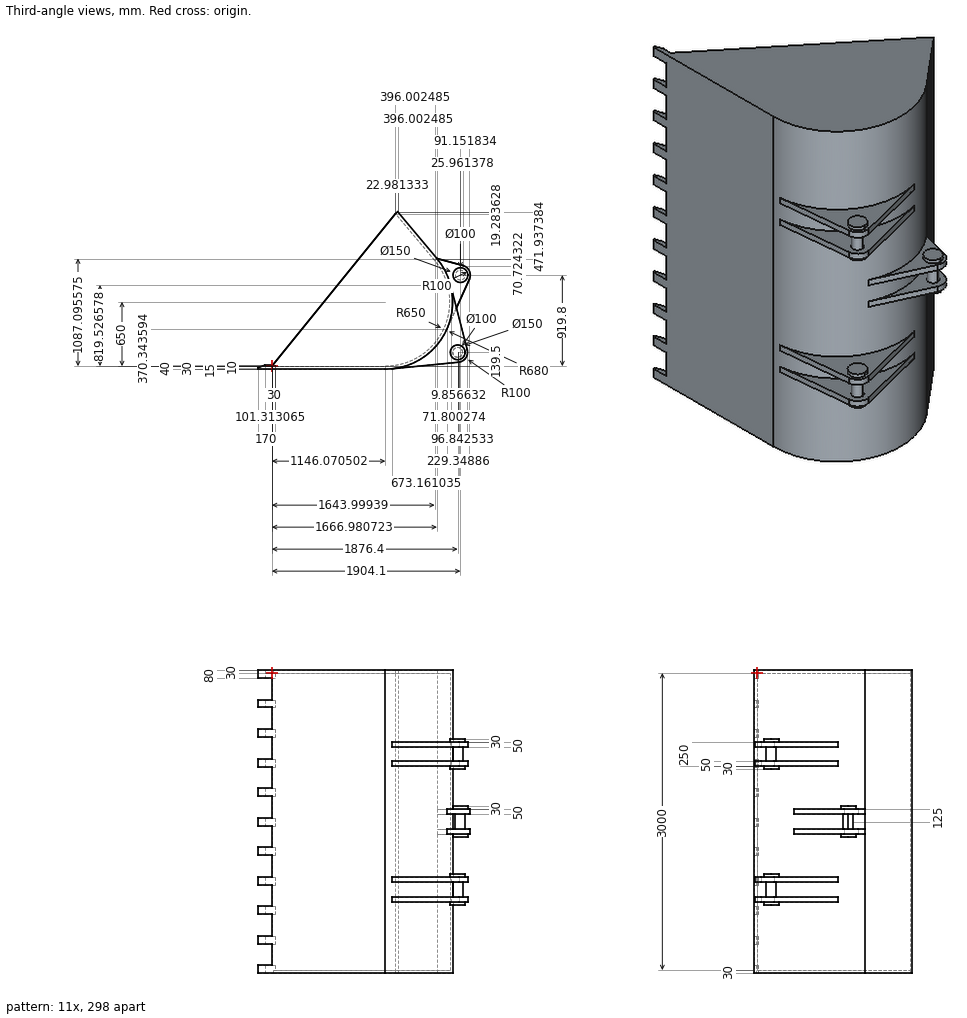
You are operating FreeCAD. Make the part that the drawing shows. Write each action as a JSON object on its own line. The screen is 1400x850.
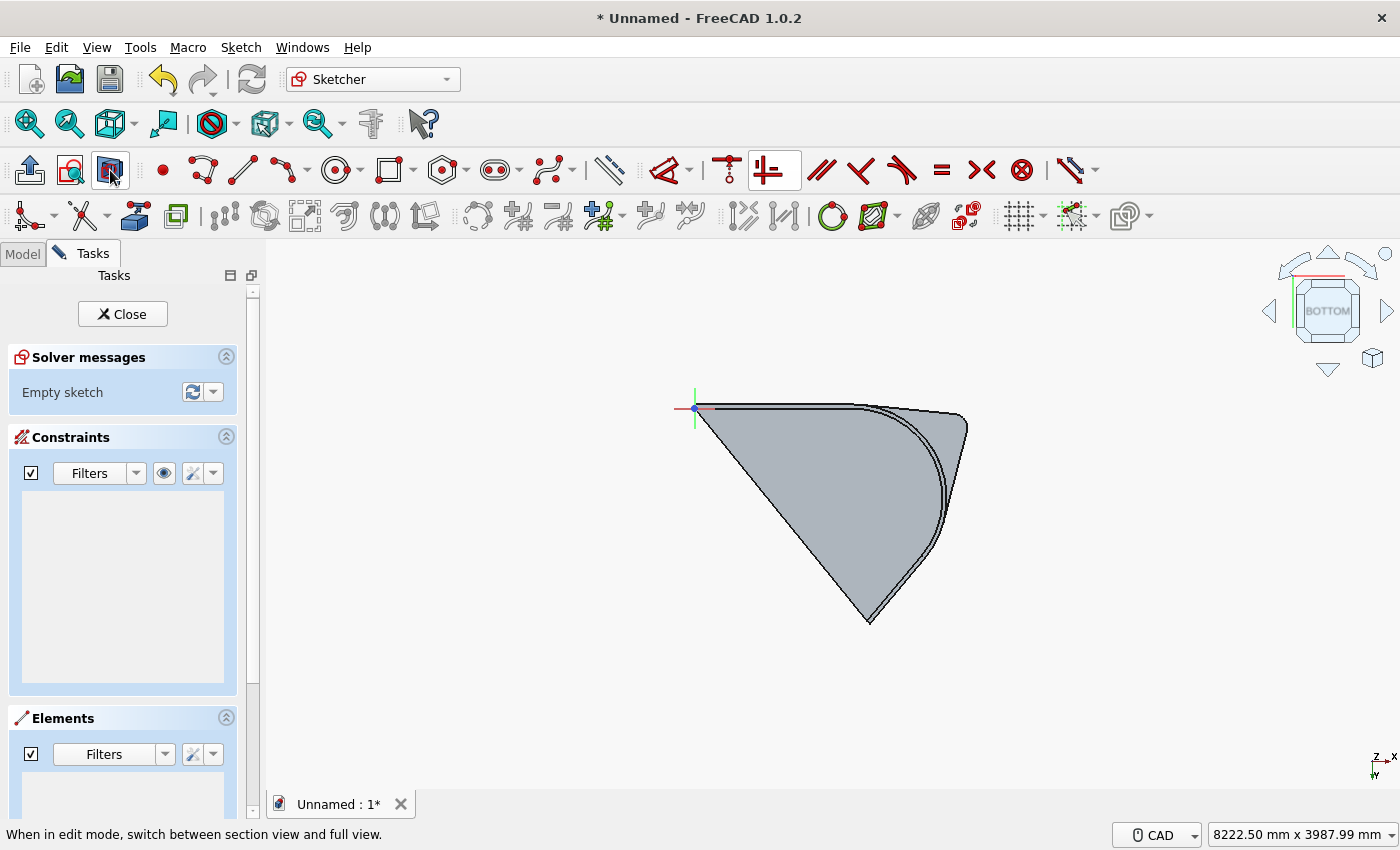
{"action": "scroll", "coordinate": [966, 422], "scroll_direction": "up", "scroll_amount": 14}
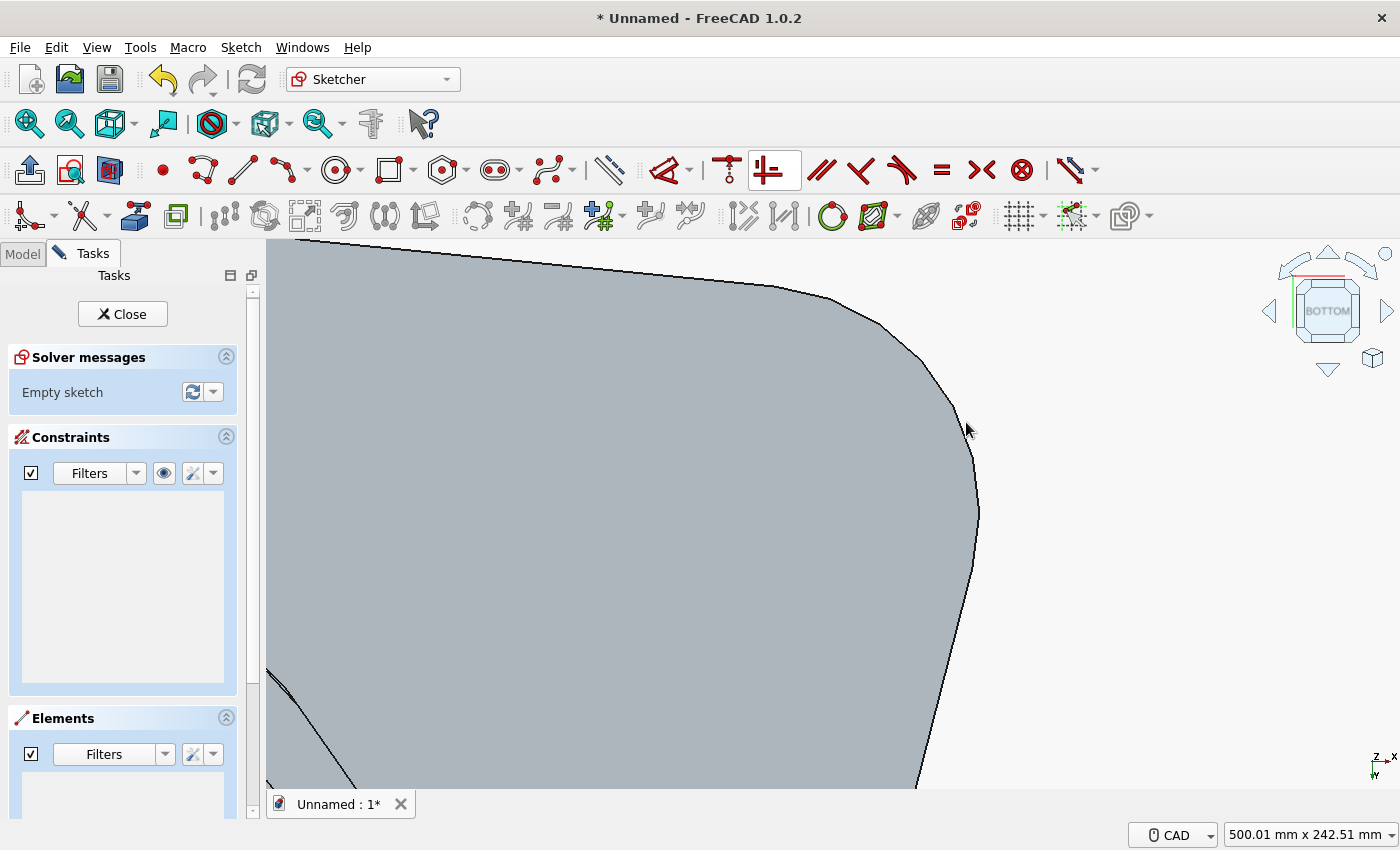
{"action": "key", "text": "g c"}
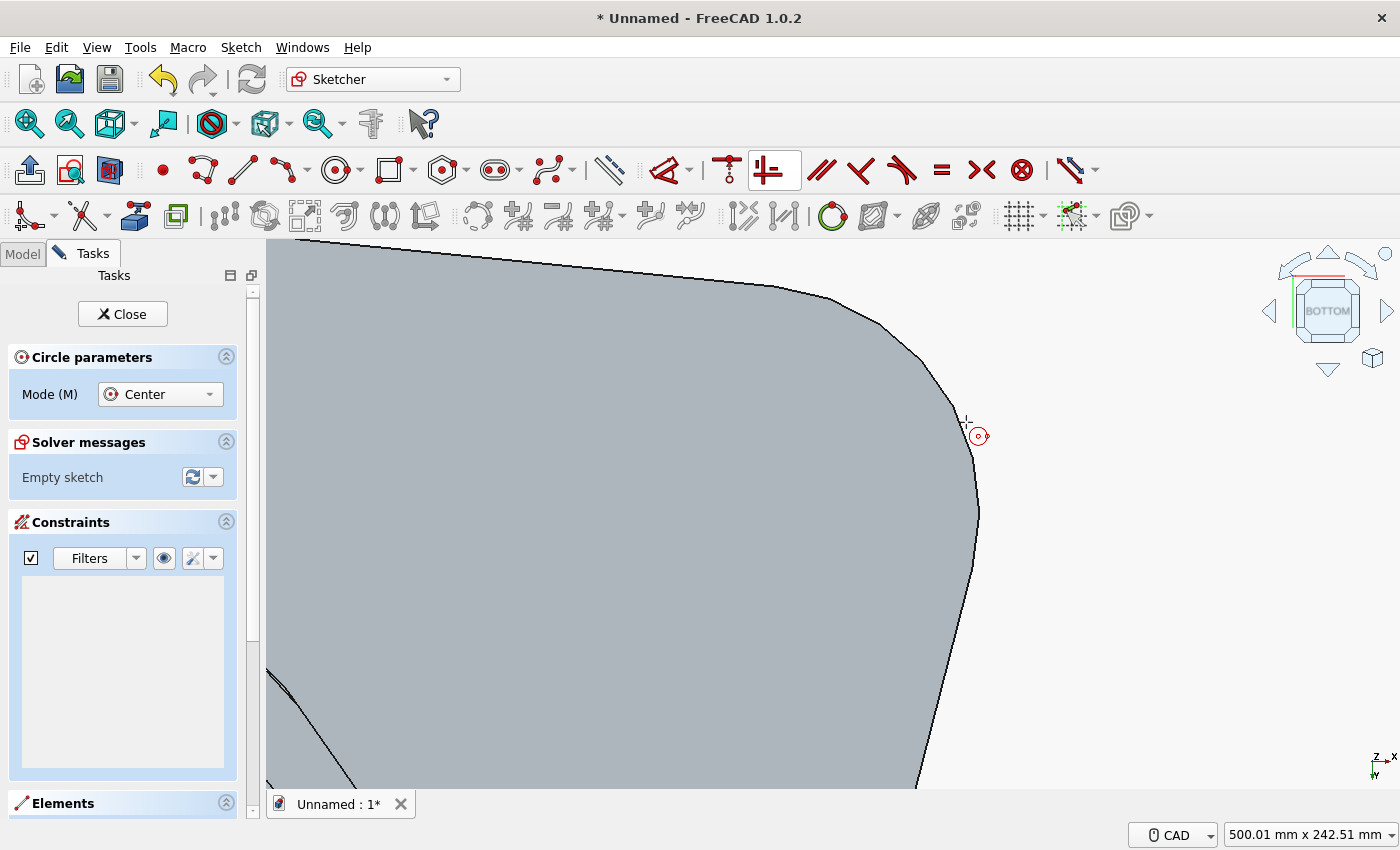
{"action": "left_click", "coordinate": [753, 512]}
{"action": "left_click", "coordinate": [873, 392]}
{"action": "key", "text": "Escape"}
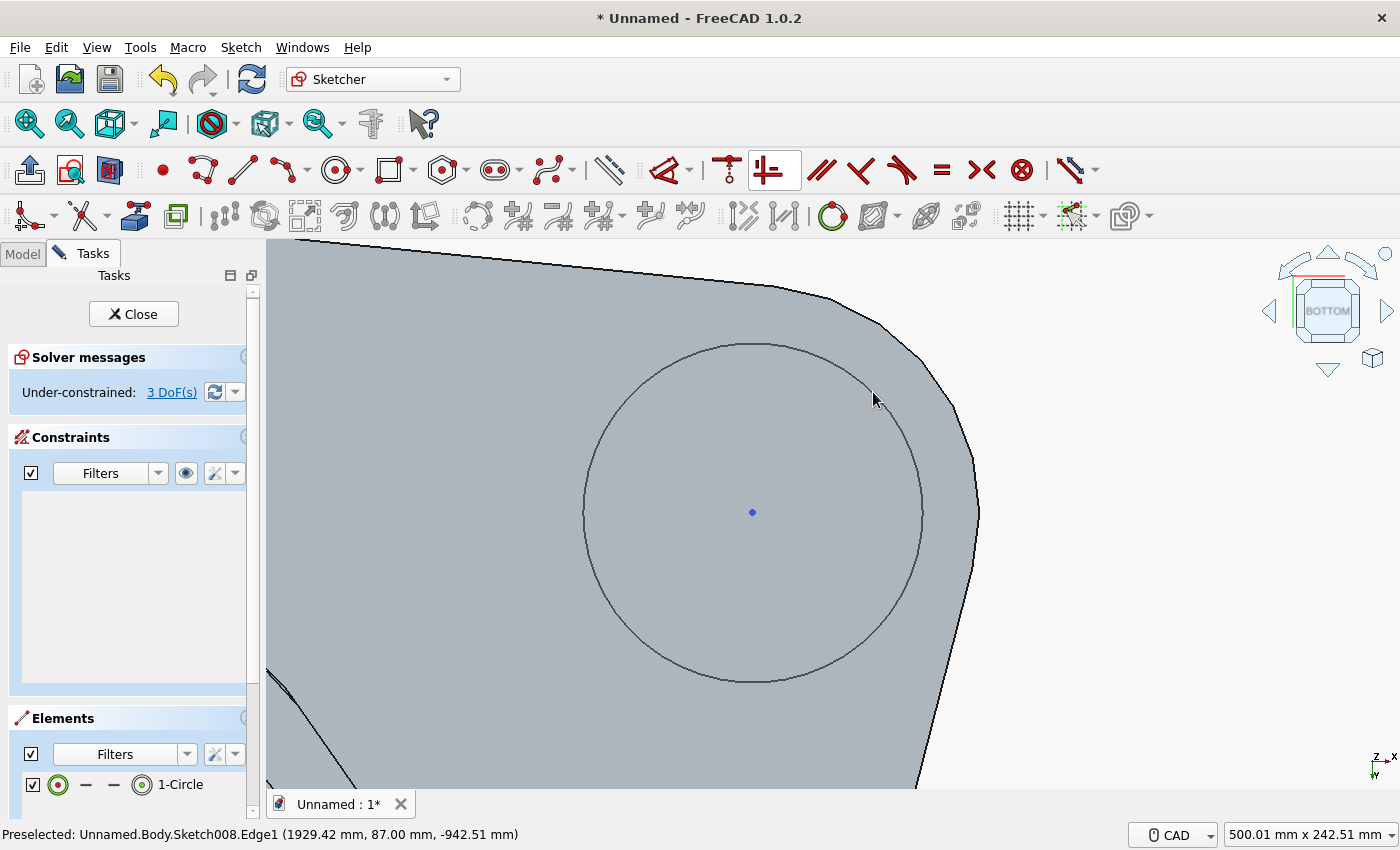
{"action": "key", "text": "d"}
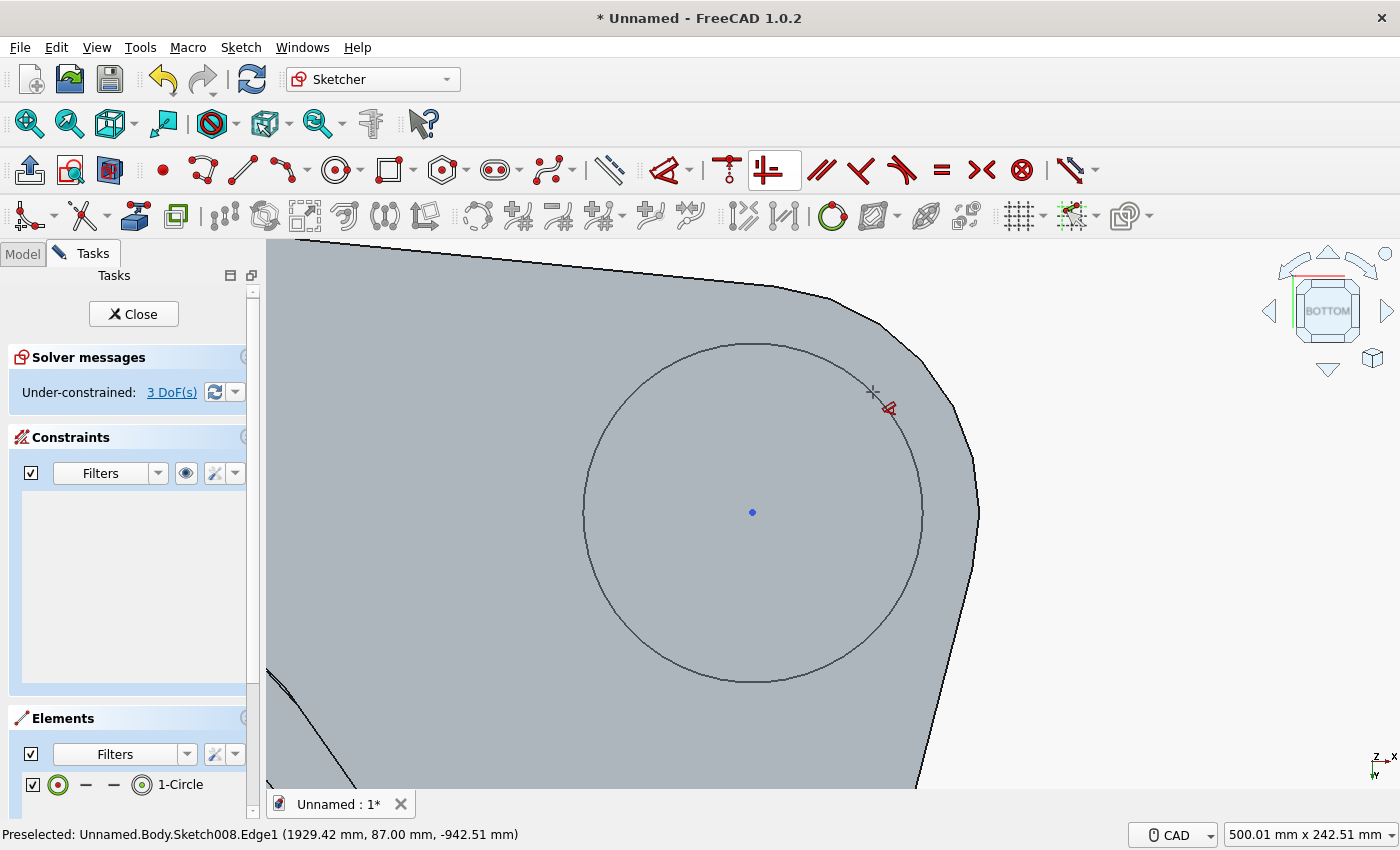
{"action": "left_click", "coordinate": [873, 393]}
{"action": "left_click", "coordinate": [896, 370]}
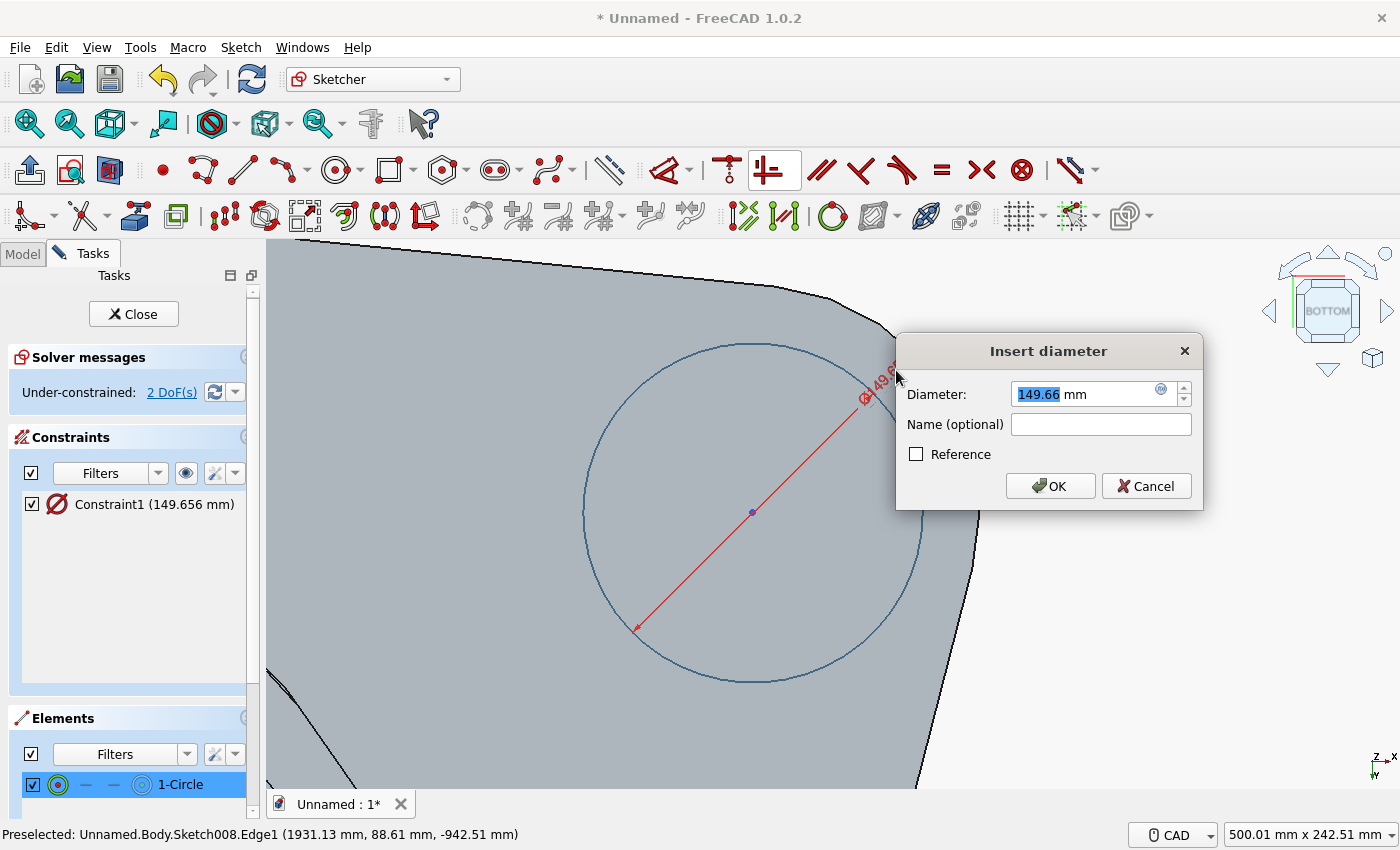
{"action": "type", "text": "150"}
{"action": "key", "text": "Return"}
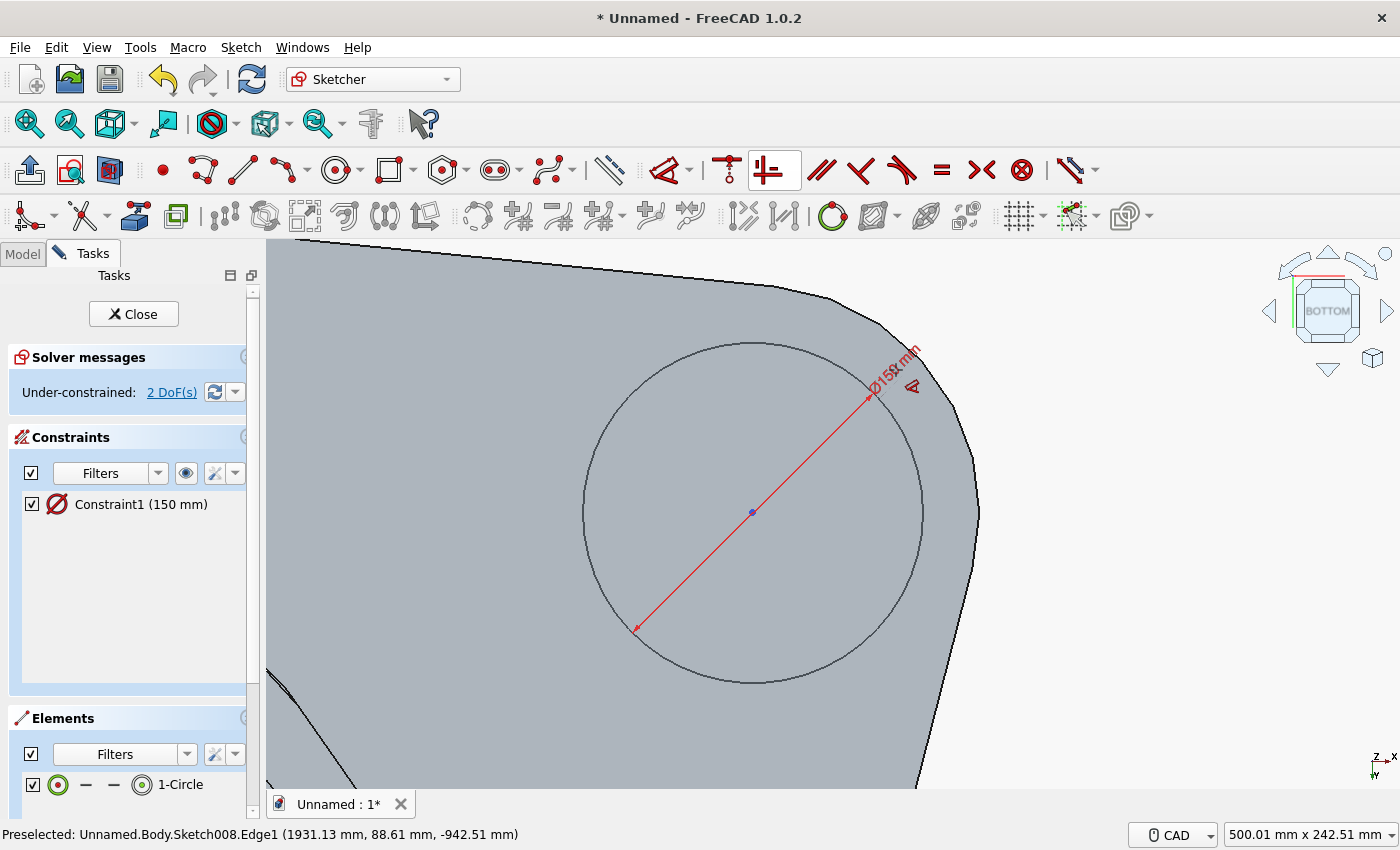
{"action": "left_click", "coordinate": [753, 513]}
{"action": "left_click", "coordinate": [787, 390]}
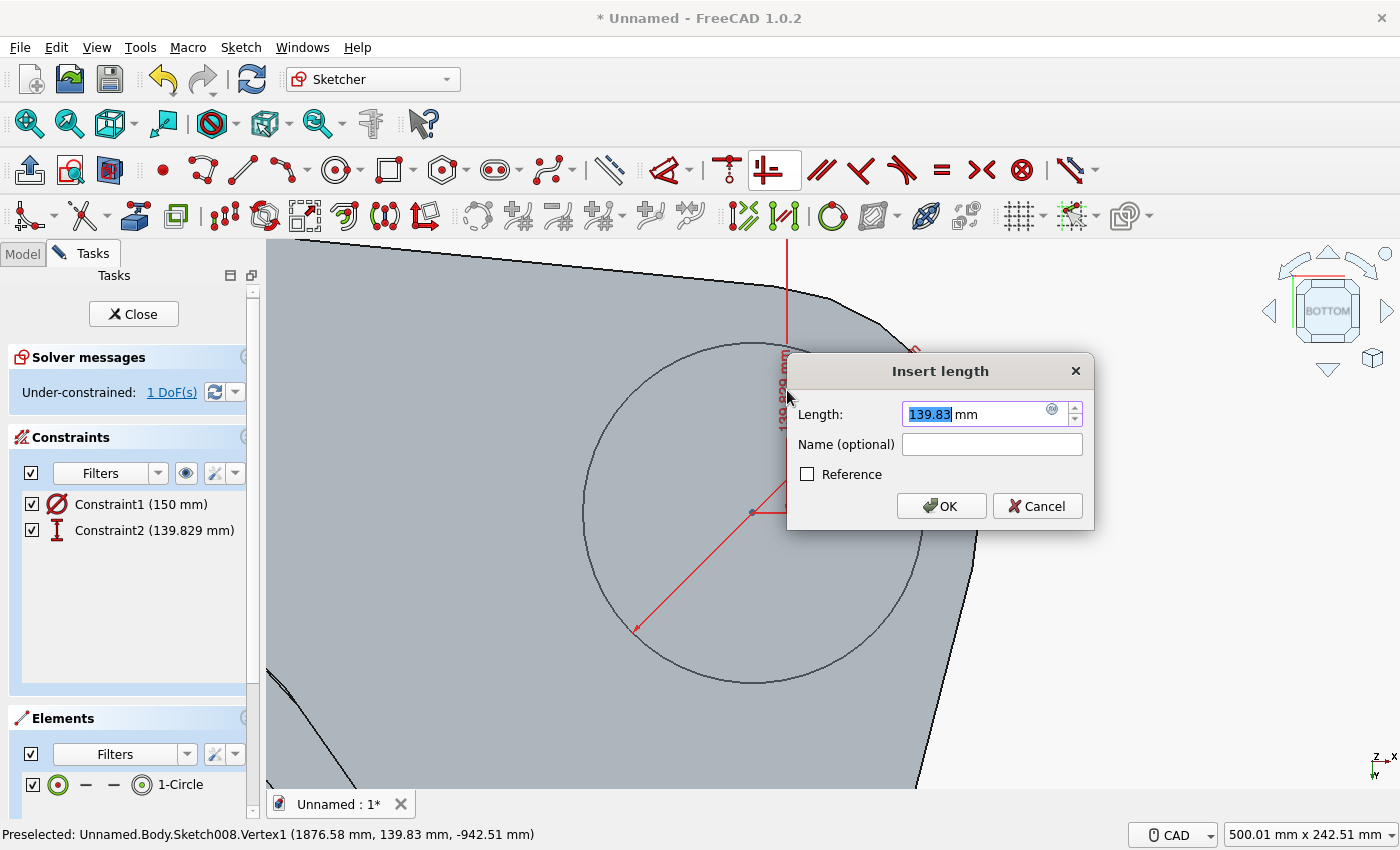
{"action": "type", "text": "139.5"}
{"action": "key", "text": "Return"}